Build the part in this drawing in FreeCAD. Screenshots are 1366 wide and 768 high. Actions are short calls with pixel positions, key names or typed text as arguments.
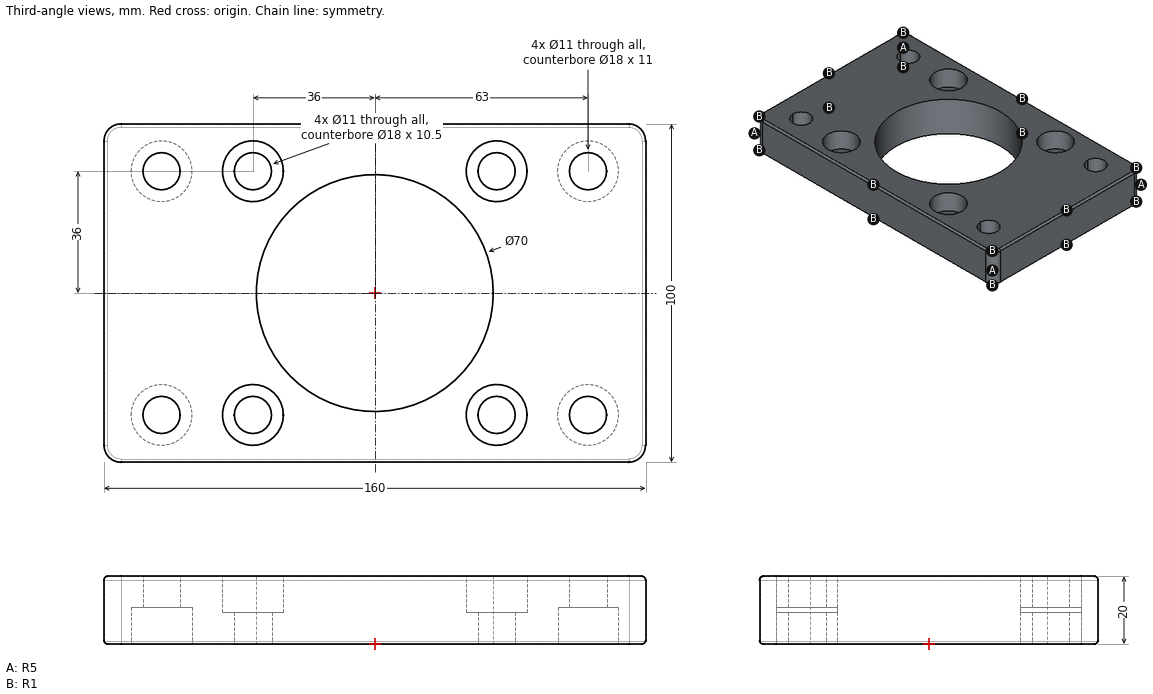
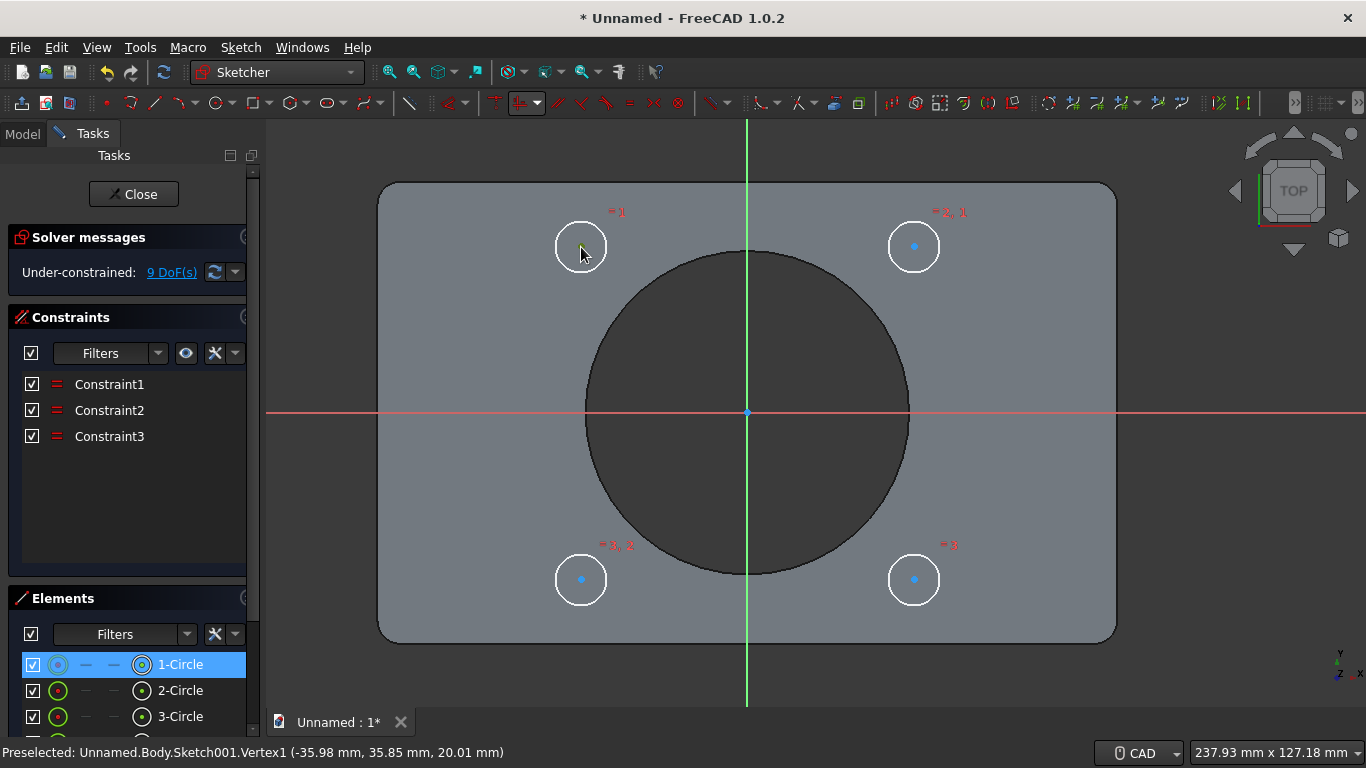
click(914, 247)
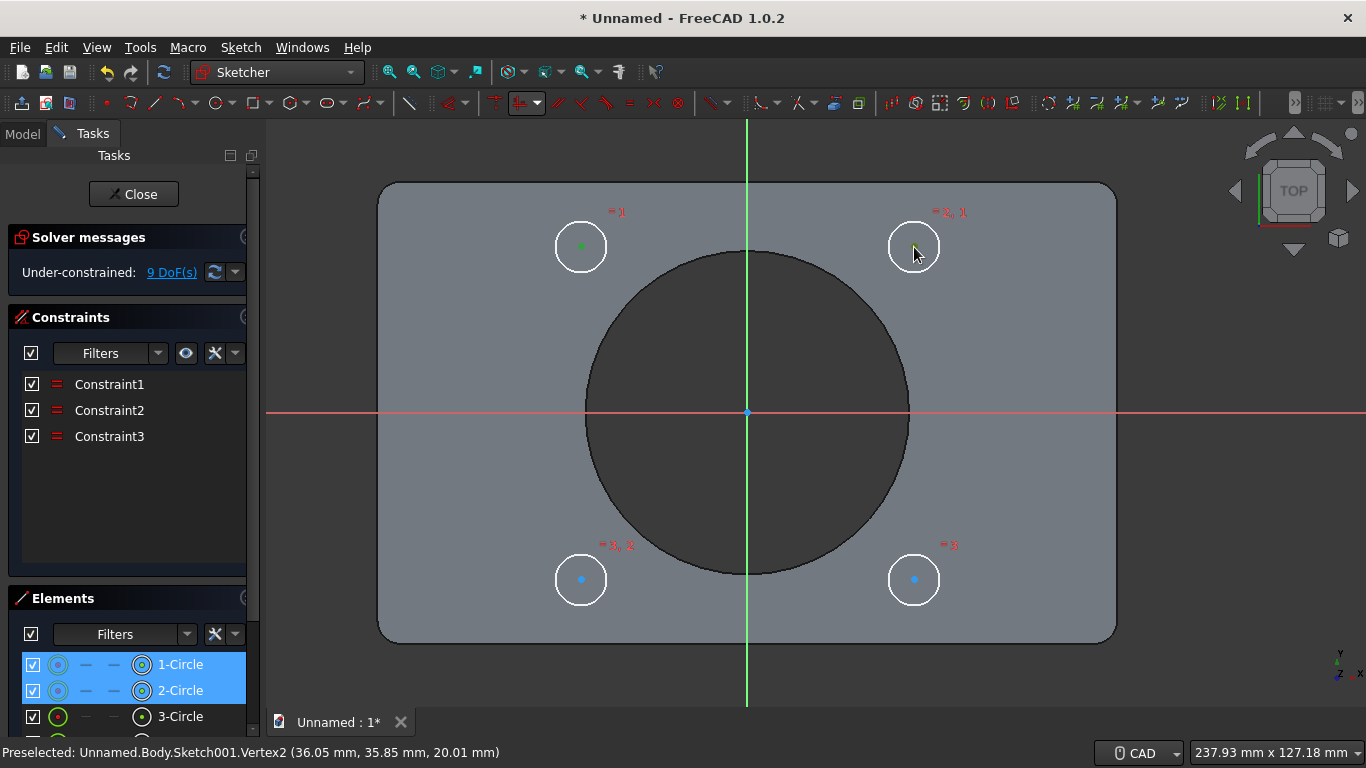
click(747, 641)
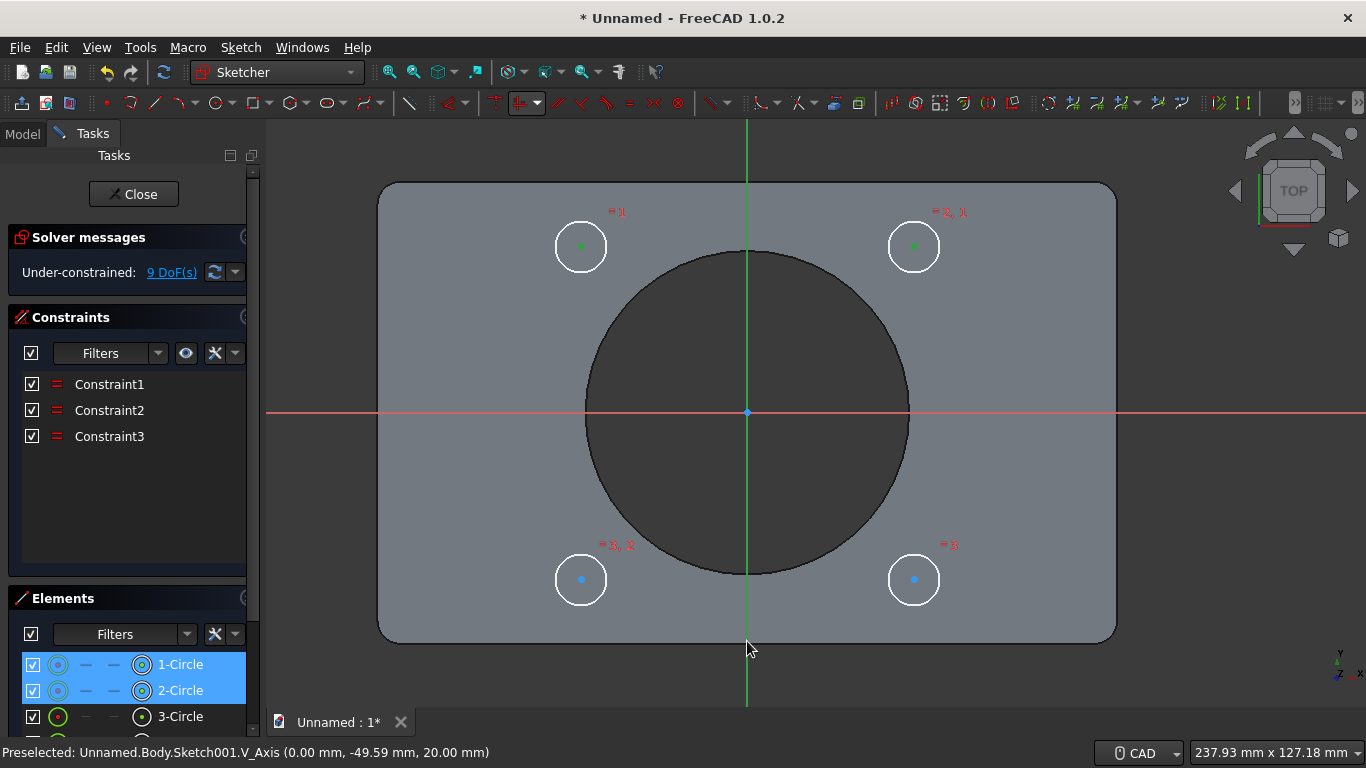
click(654, 104)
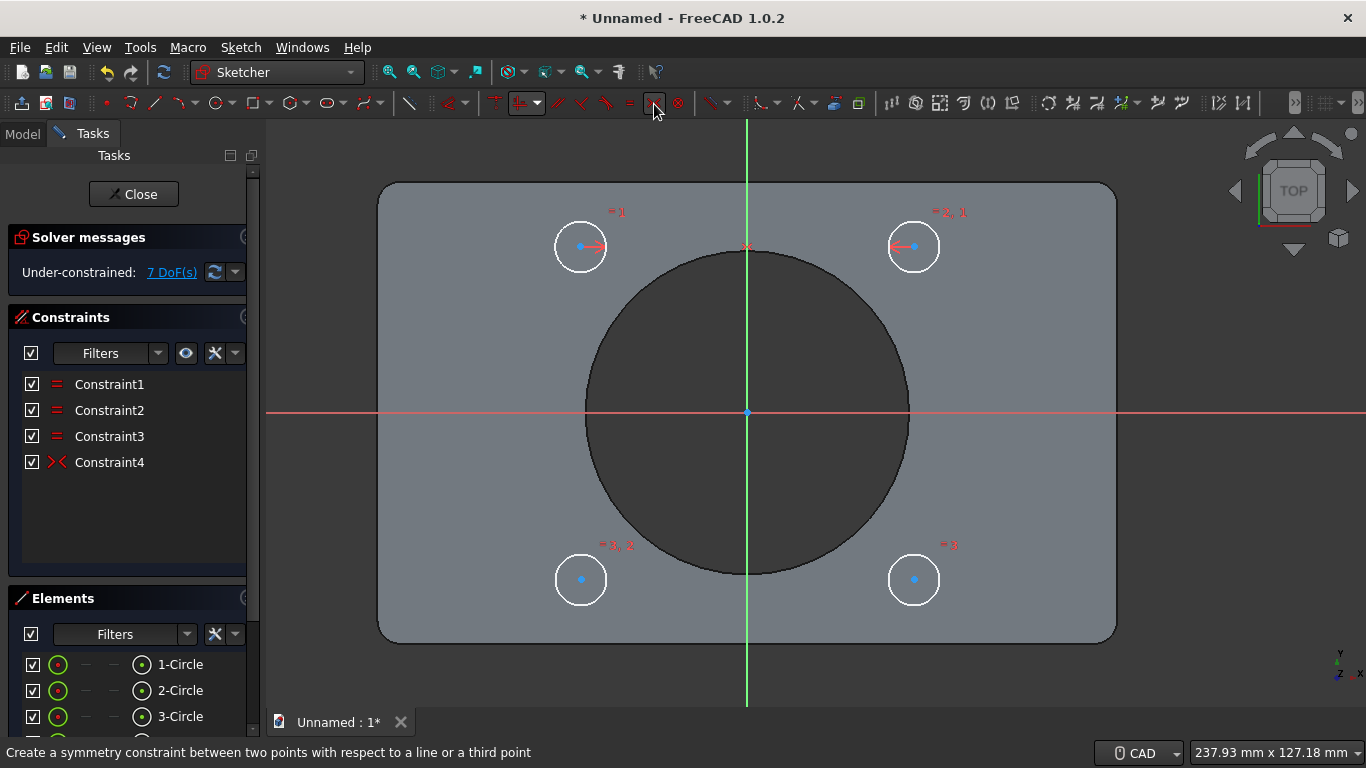
click(581, 247)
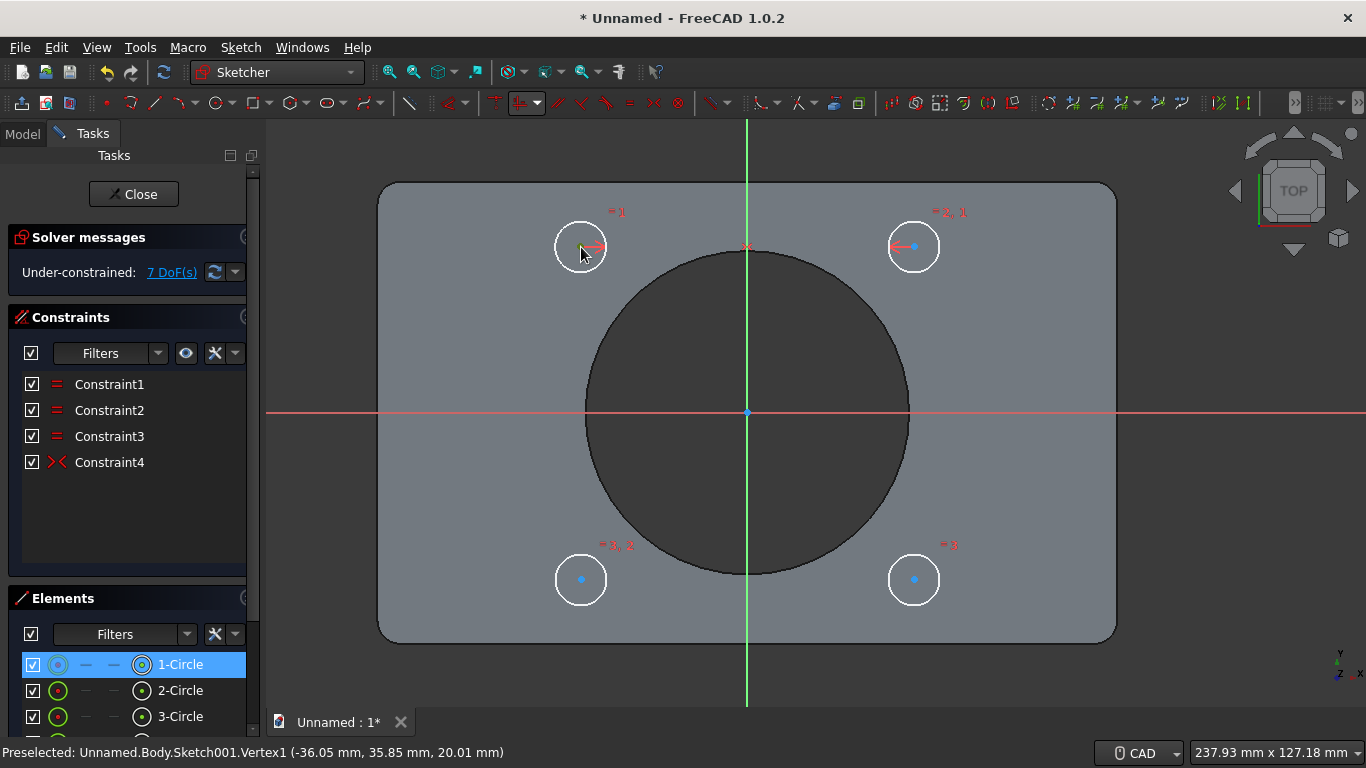
click(581, 580)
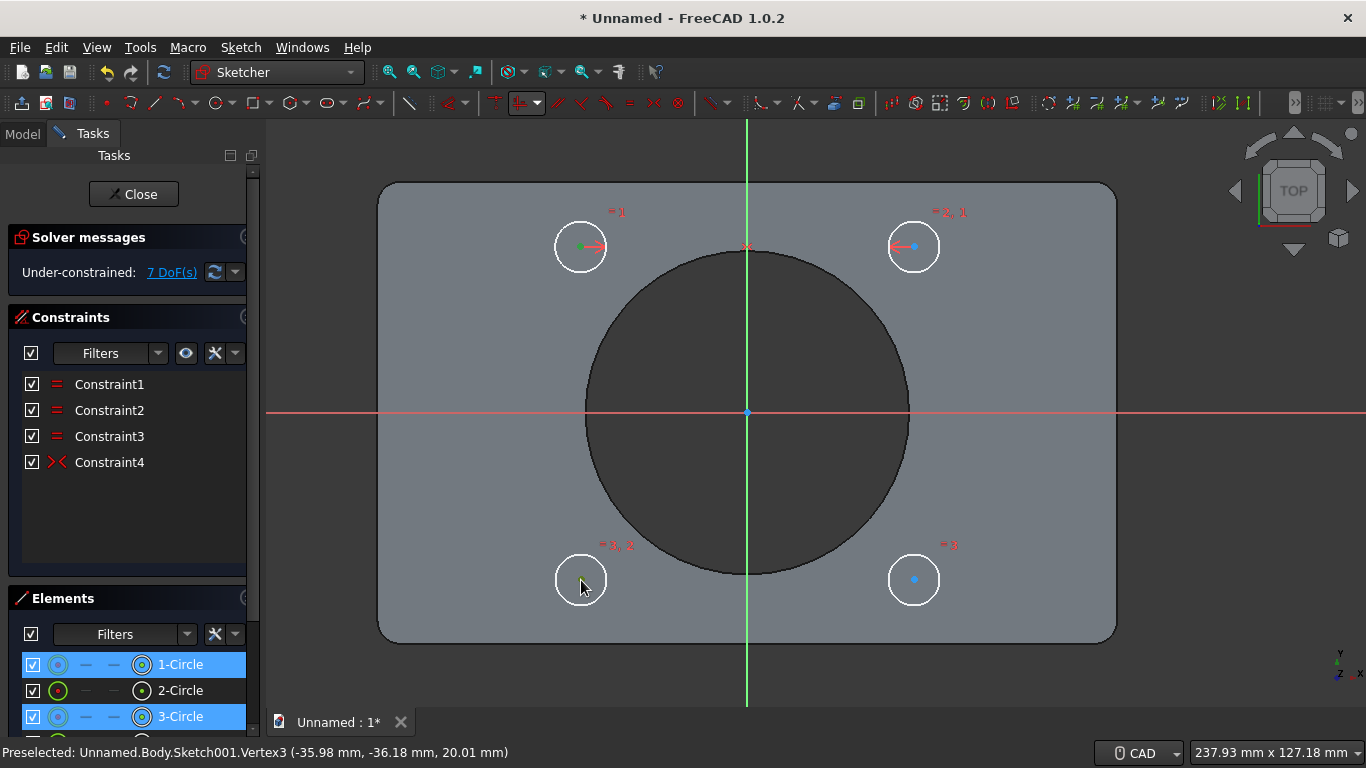
click(359, 413)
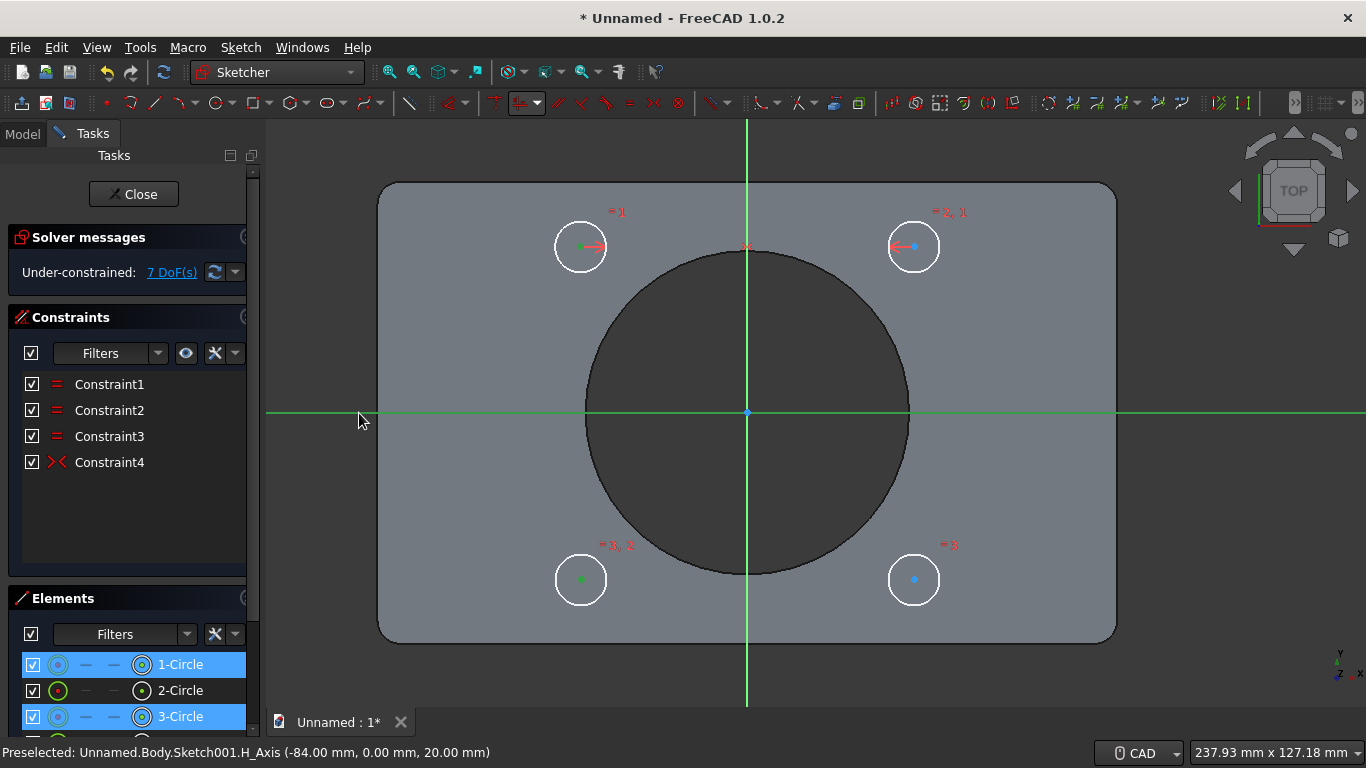
click(654, 104)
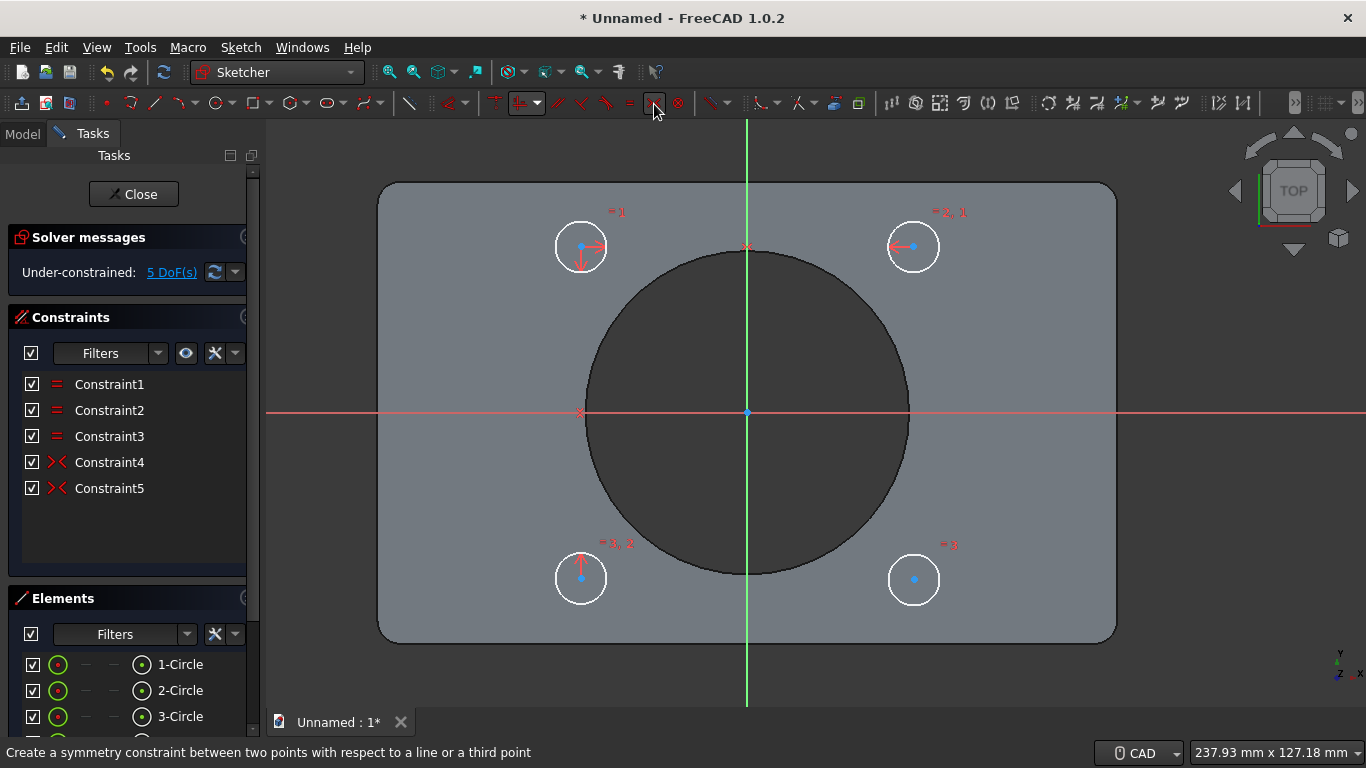
click(914, 247)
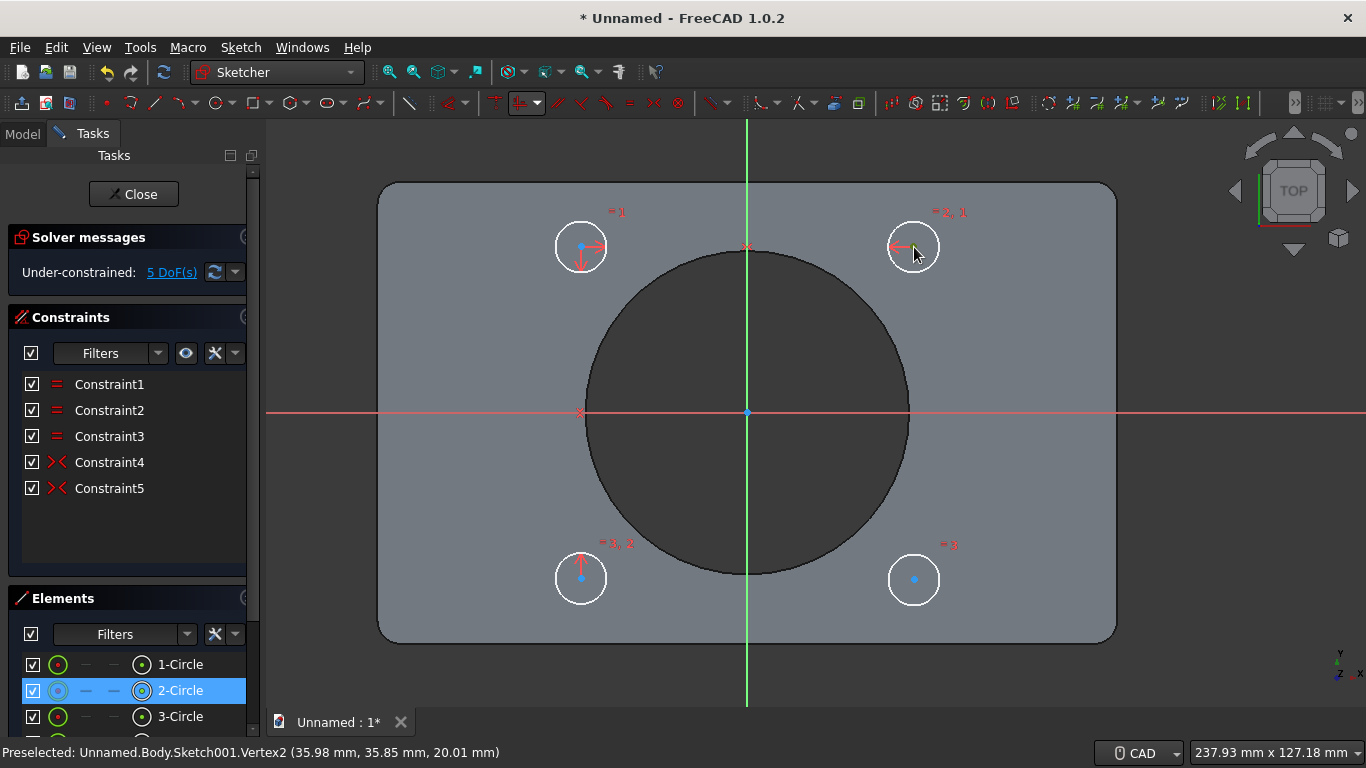
click(914, 580)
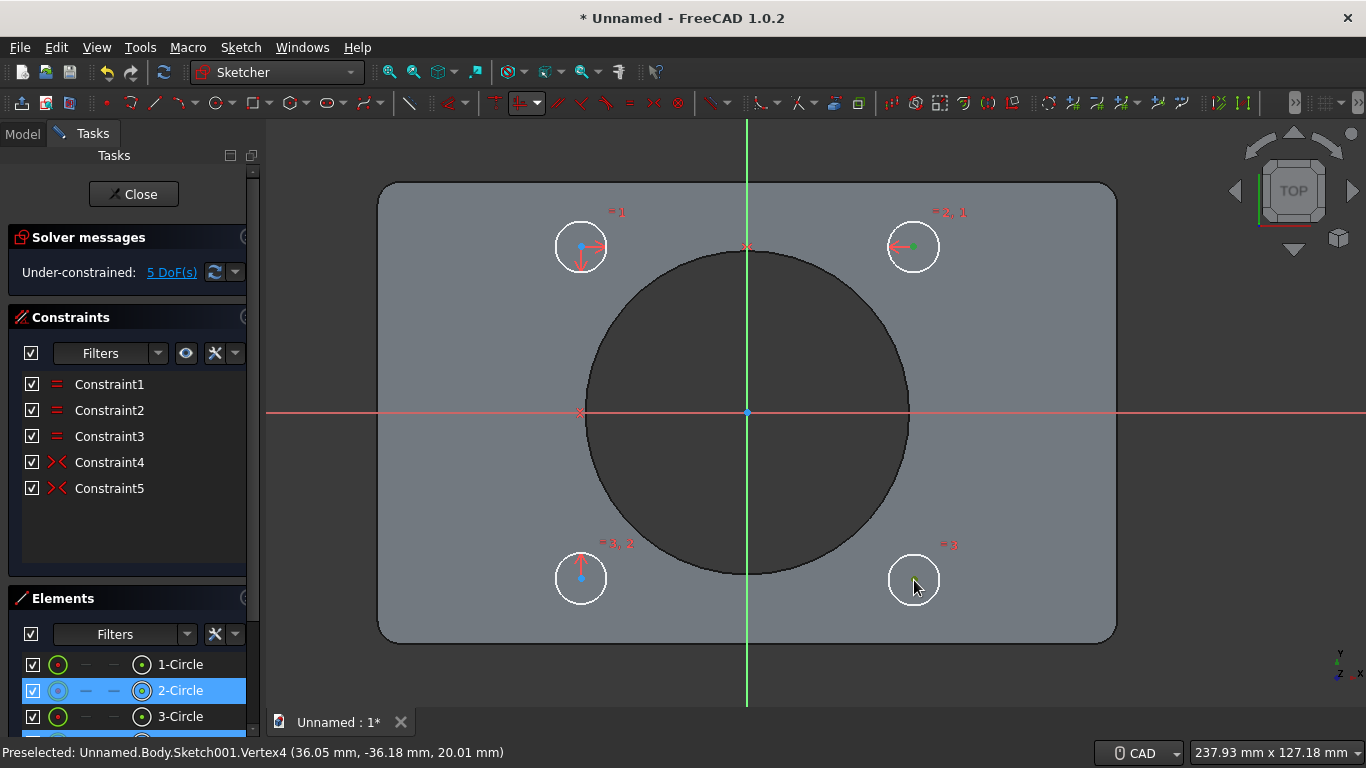
click(359, 413)